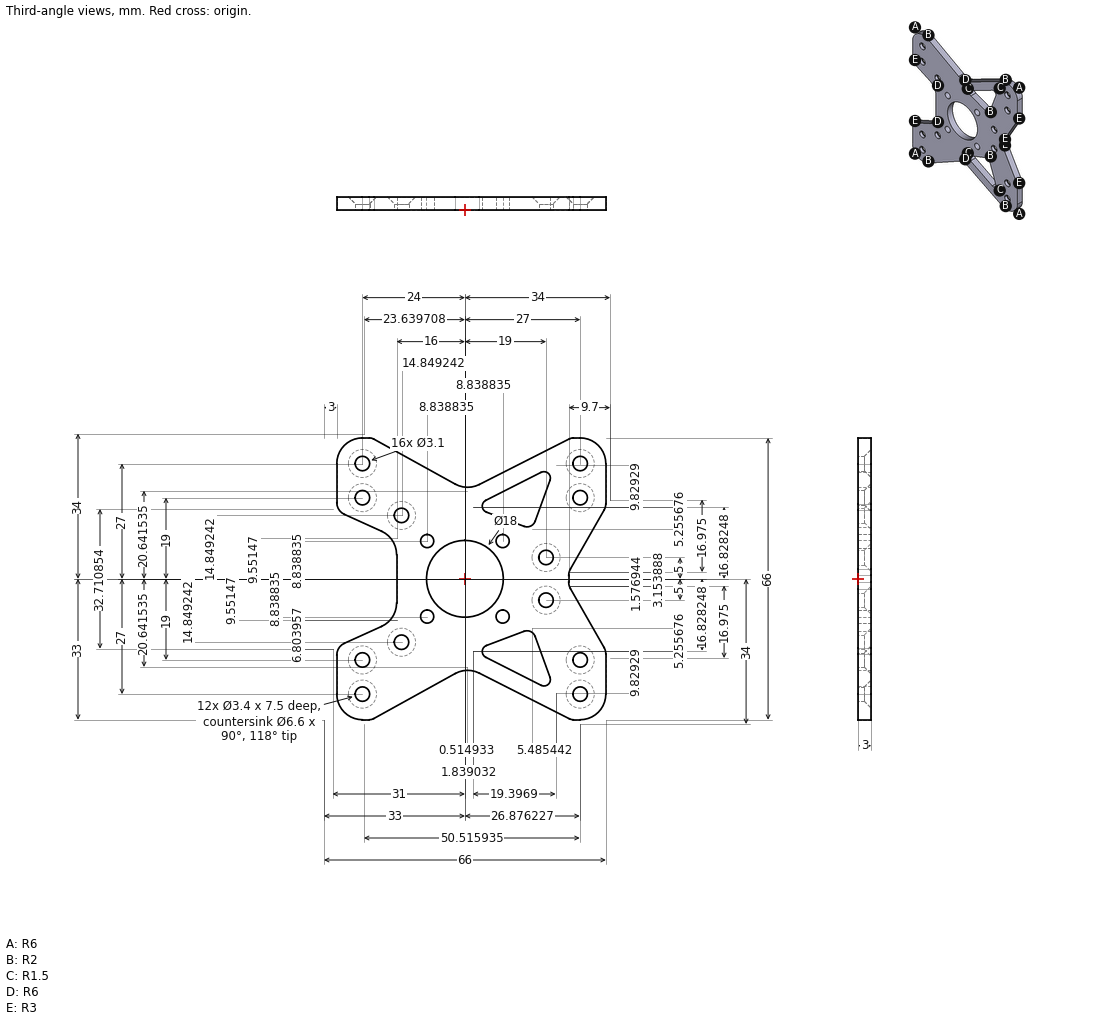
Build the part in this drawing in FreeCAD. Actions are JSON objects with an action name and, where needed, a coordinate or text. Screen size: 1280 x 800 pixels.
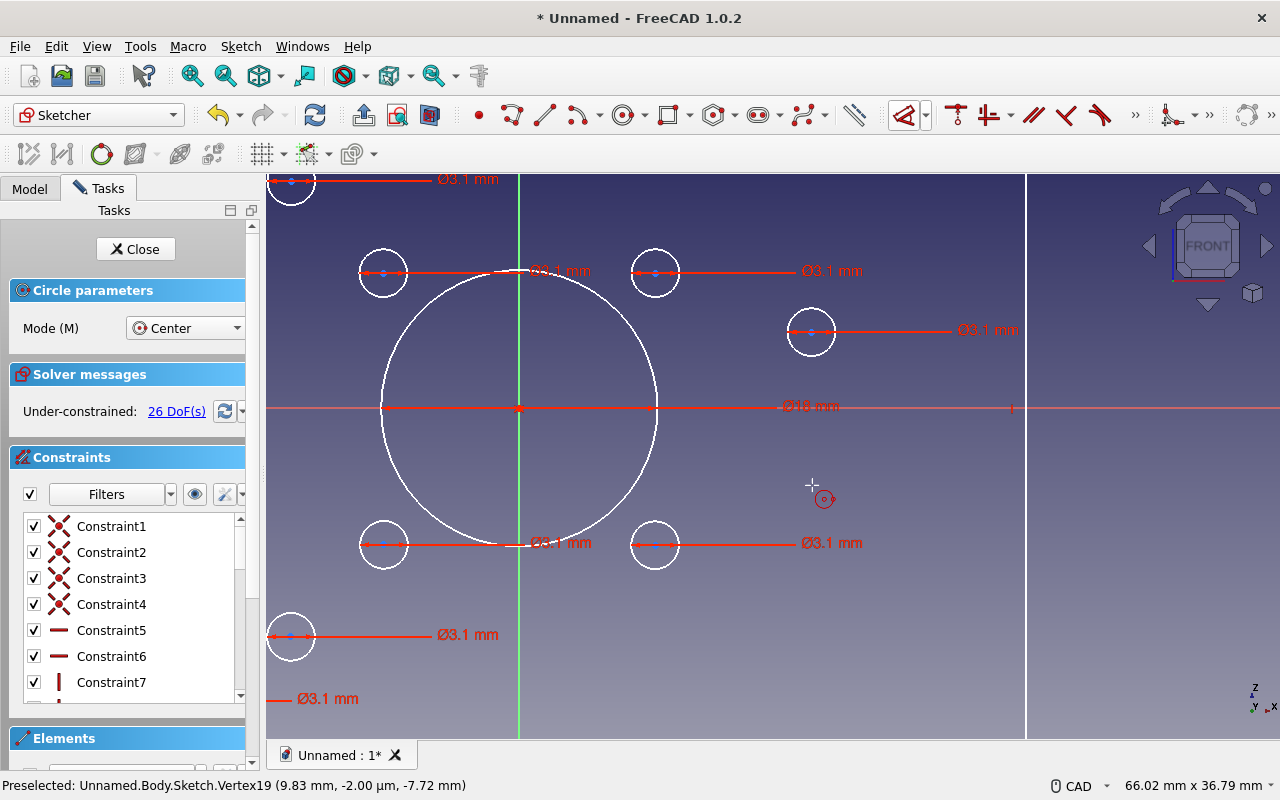
{"action": "left_click", "coordinate": [811, 485]}
{"action": "mouse_move", "coordinate": [828, 468]}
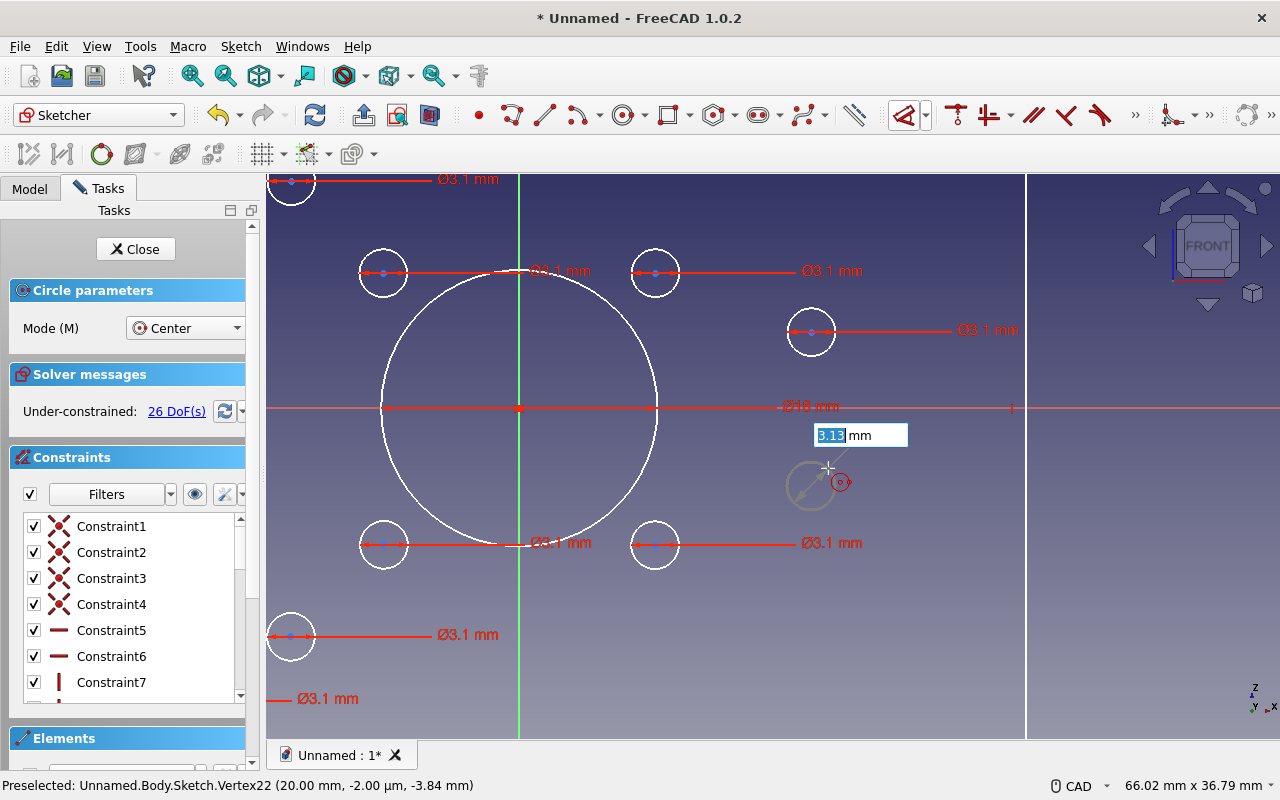
{"action": "type", "text": "3.1"}
{"action": "key", "text": "Return"}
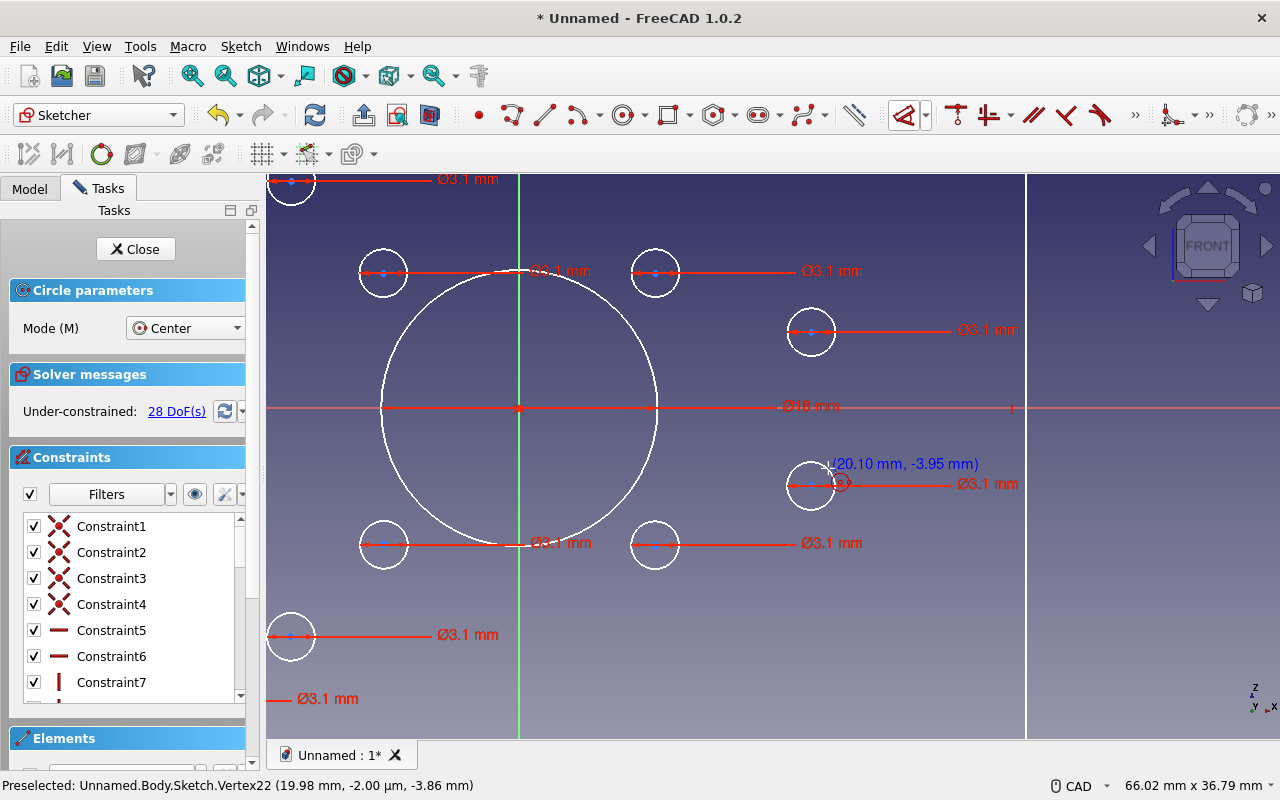
{"action": "left_click", "coordinate": [934, 700]}
{"action": "mouse_move", "coordinate": [951, 683]}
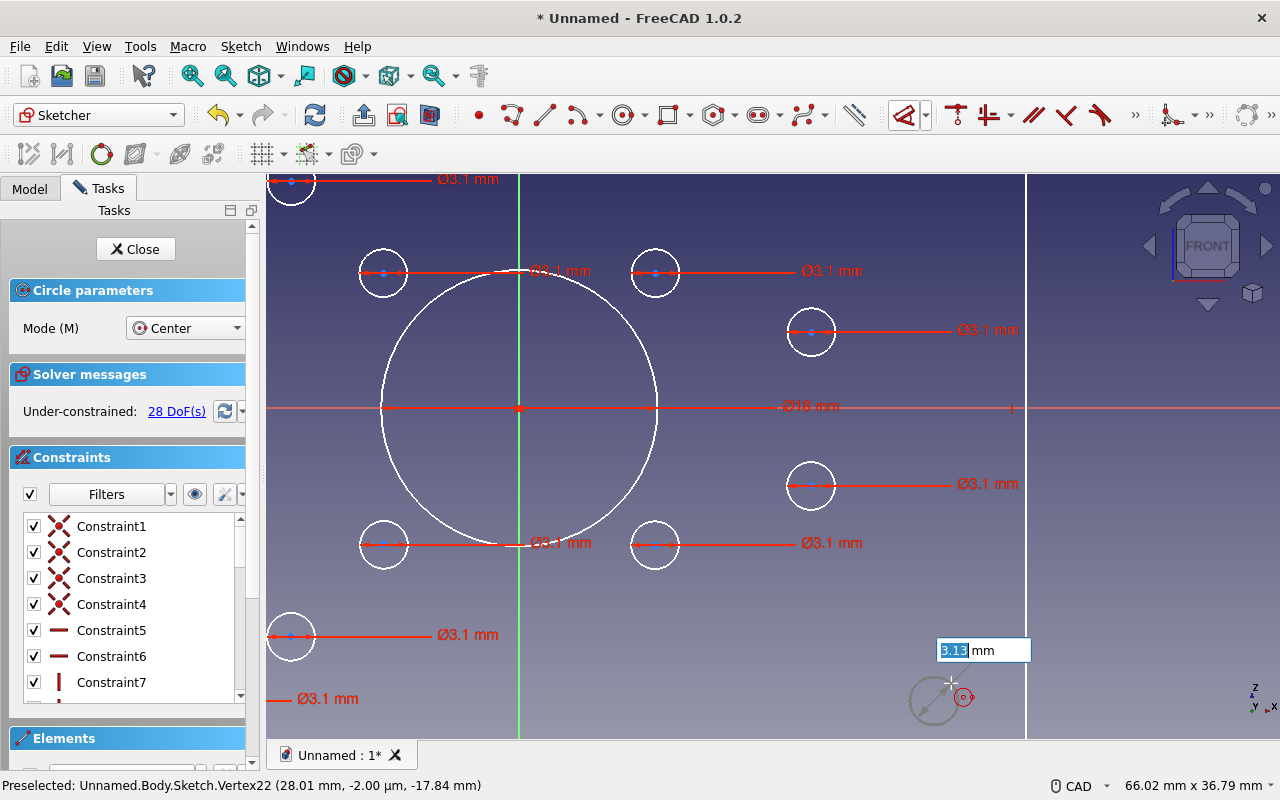
{"action": "type", "text": "3.1"}
{"action": "key", "text": "Return"}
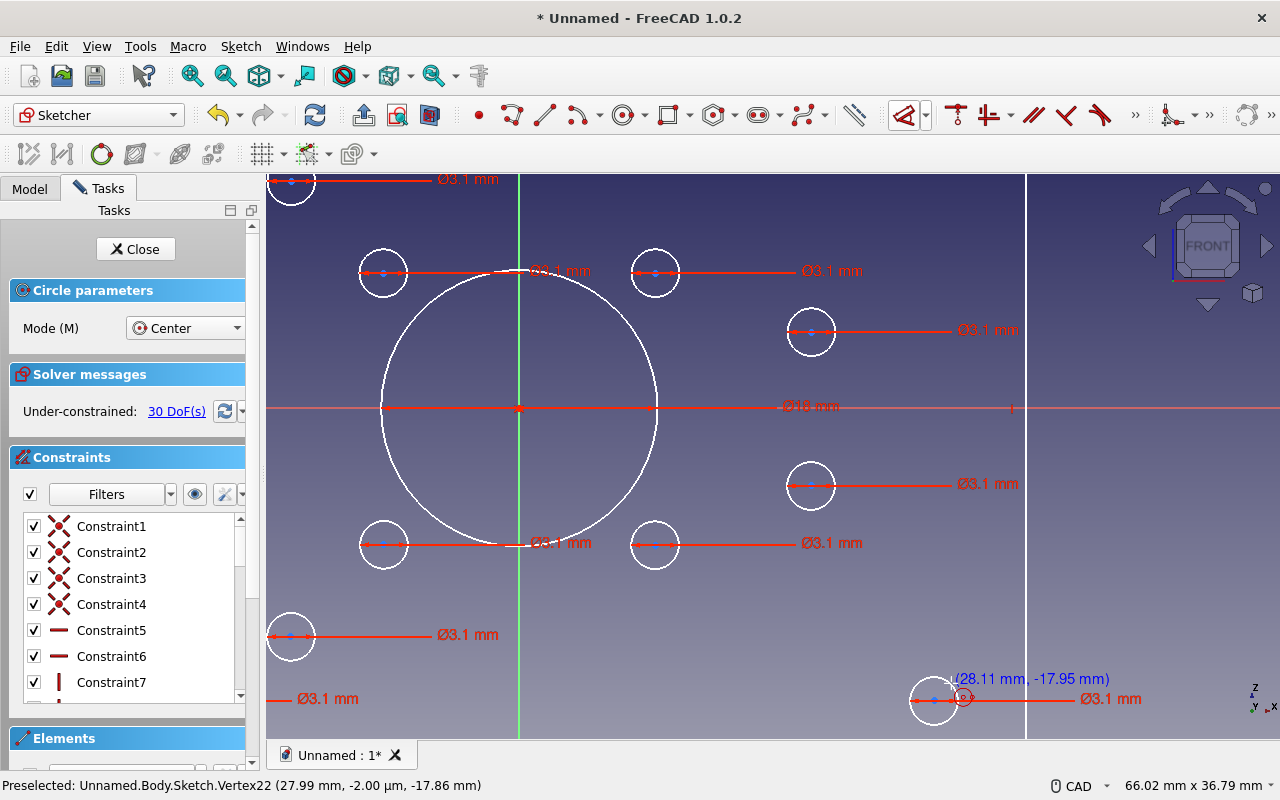
{"action": "scroll", "coordinate": [812, 485], "scroll_direction": "down", "scroll_amount": 5}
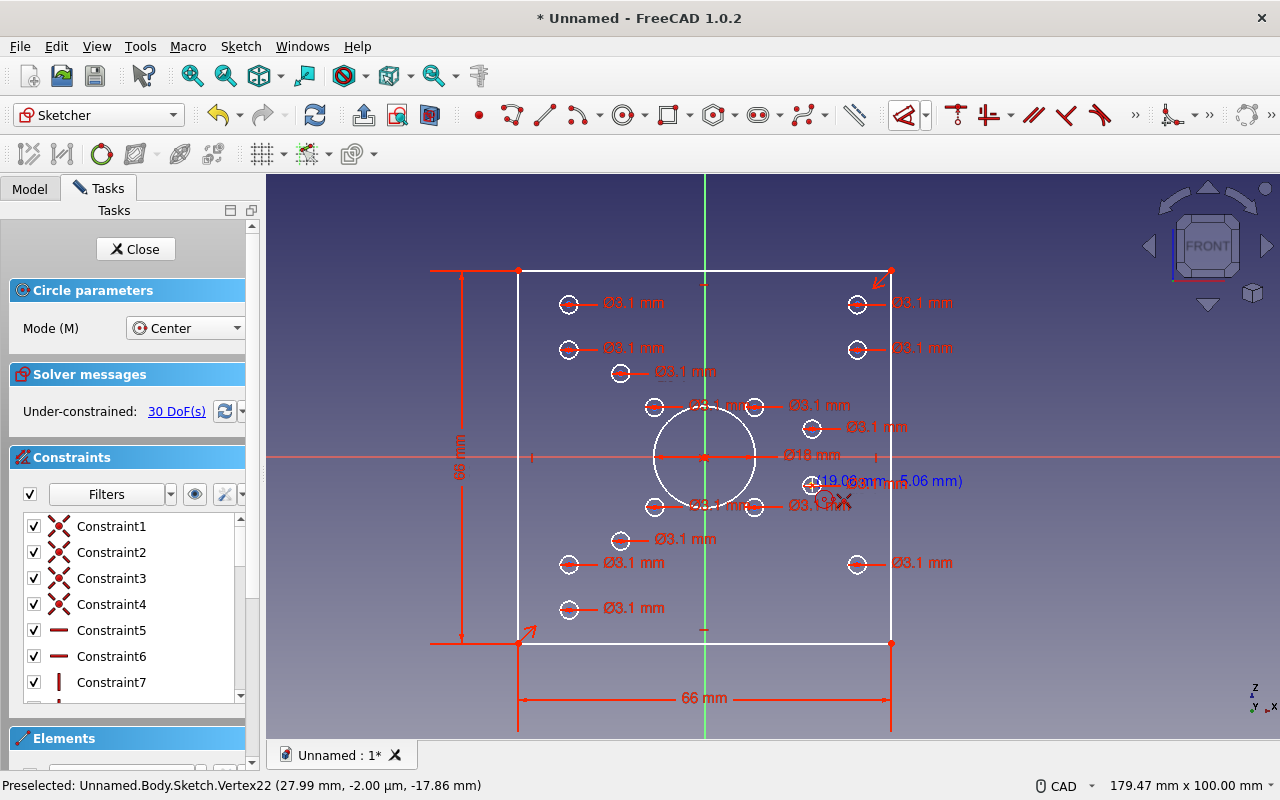
{"action": "scroll", "coordinate": [857, 610], "scroll_direction": "up", "scroll_amount": 5}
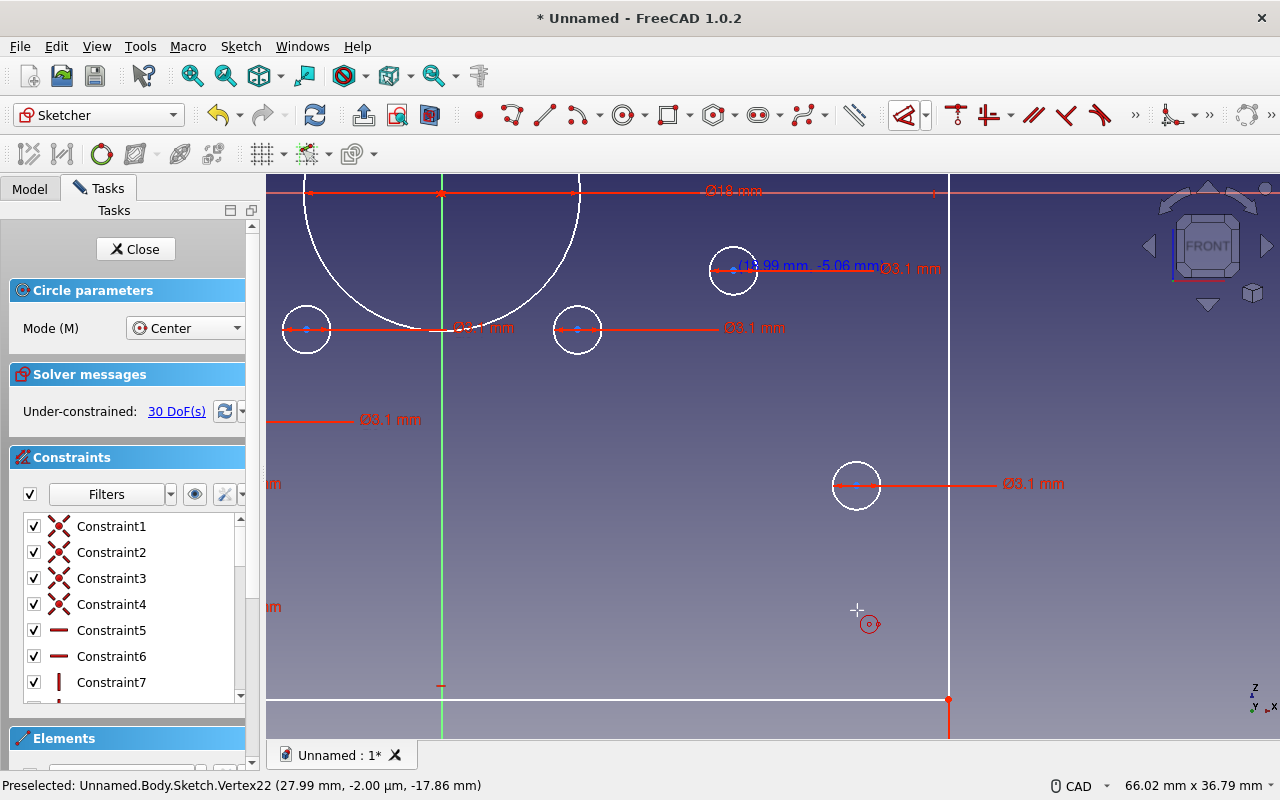
{"action": "left_click", "coordinate": [857, 608]}
{"action": "mouse_move", "coordinate": [873, 591]}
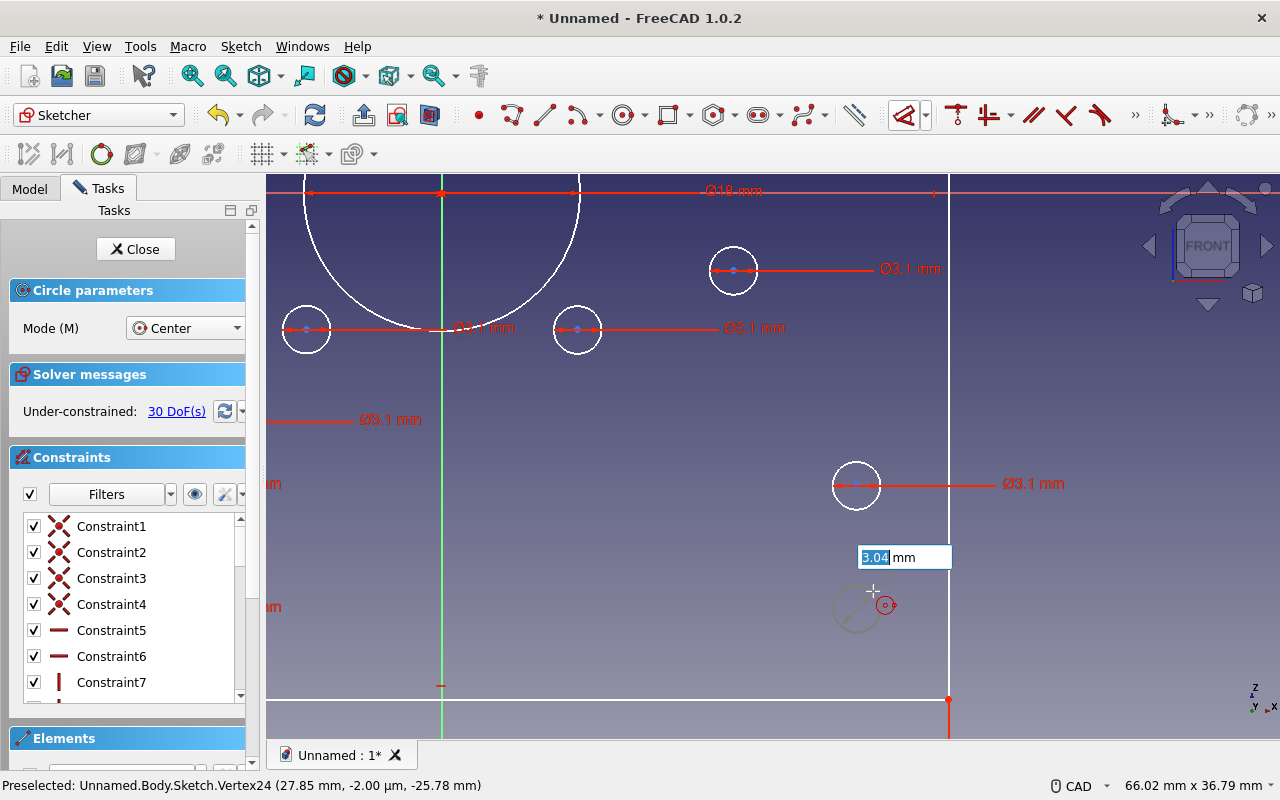
{"action": "type", "text": "3.1"}
{"action": "key", "text": "Return"}
{"action": "key", "text": "Escape"}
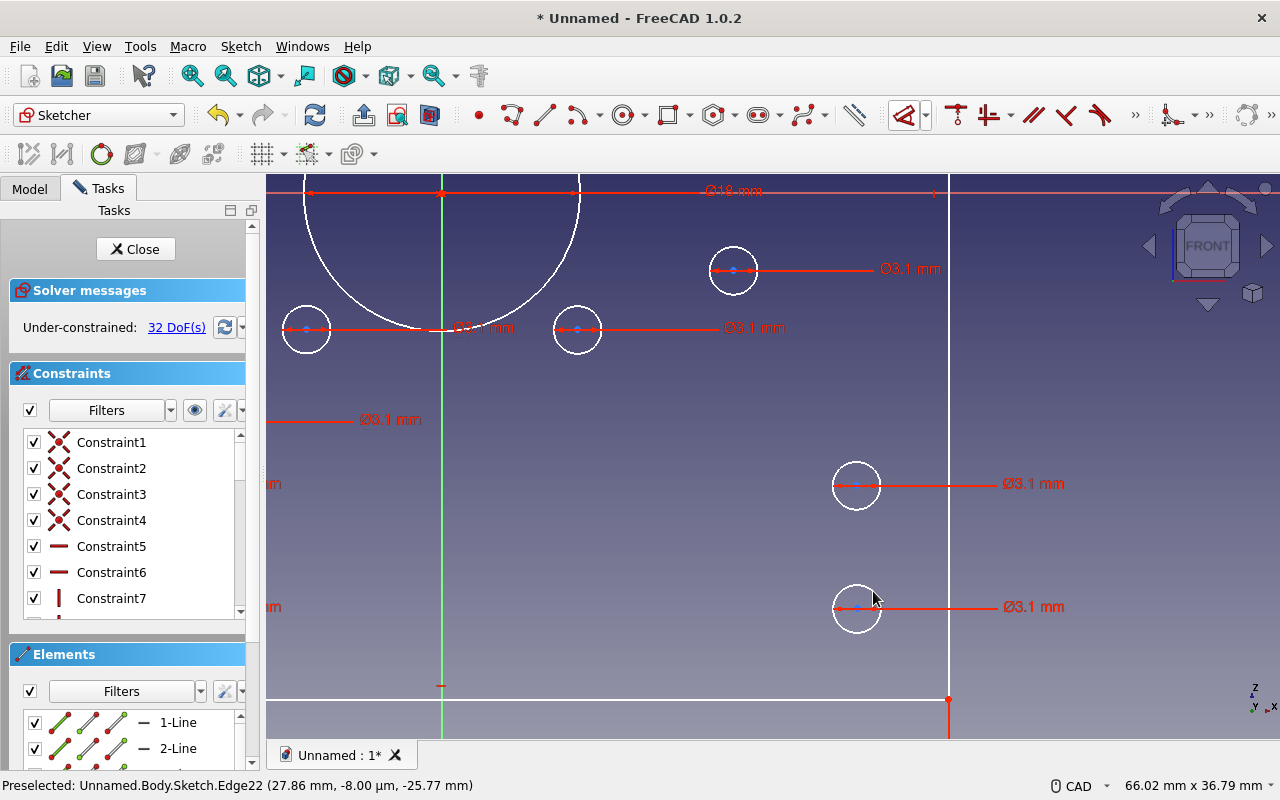
{"action": "scroll", "coordinate": [857, 610], "scroll_direction": "down", "scroll_amount": 5}